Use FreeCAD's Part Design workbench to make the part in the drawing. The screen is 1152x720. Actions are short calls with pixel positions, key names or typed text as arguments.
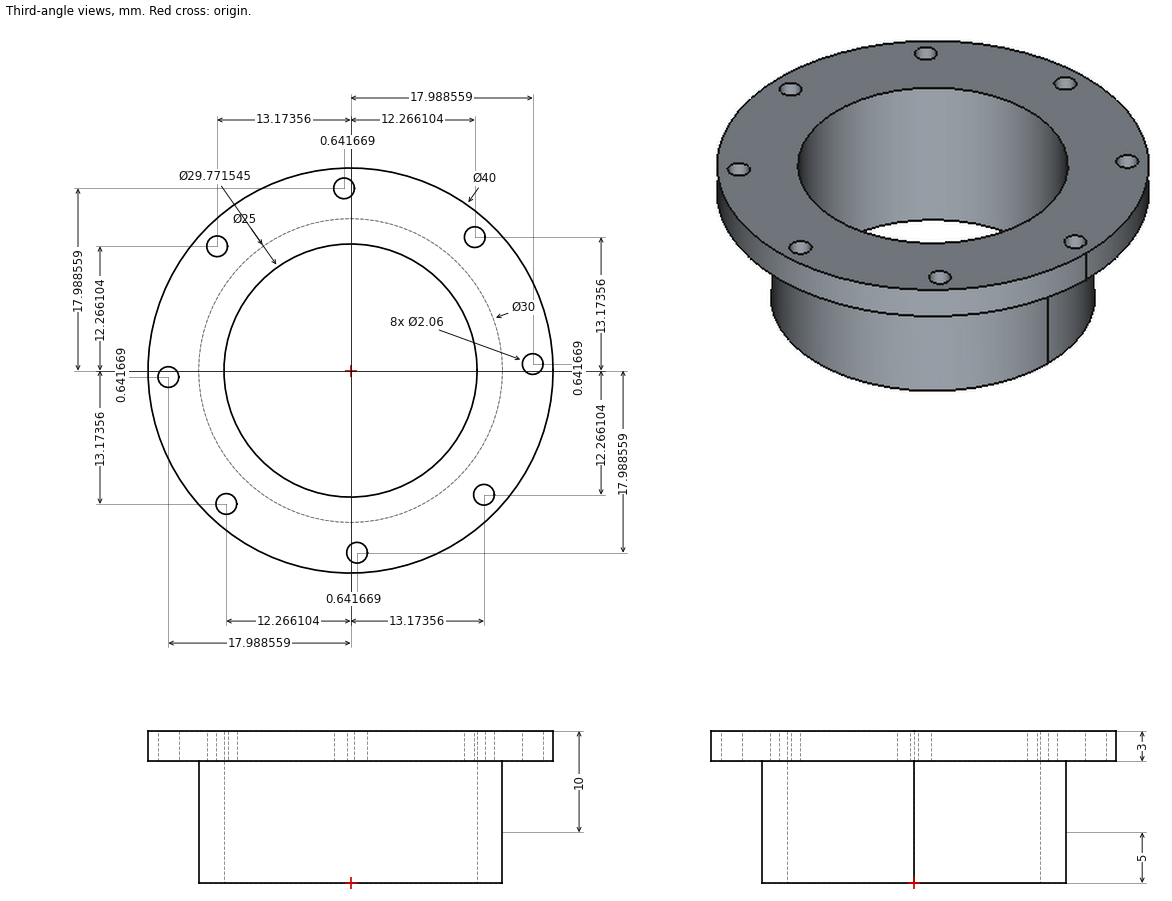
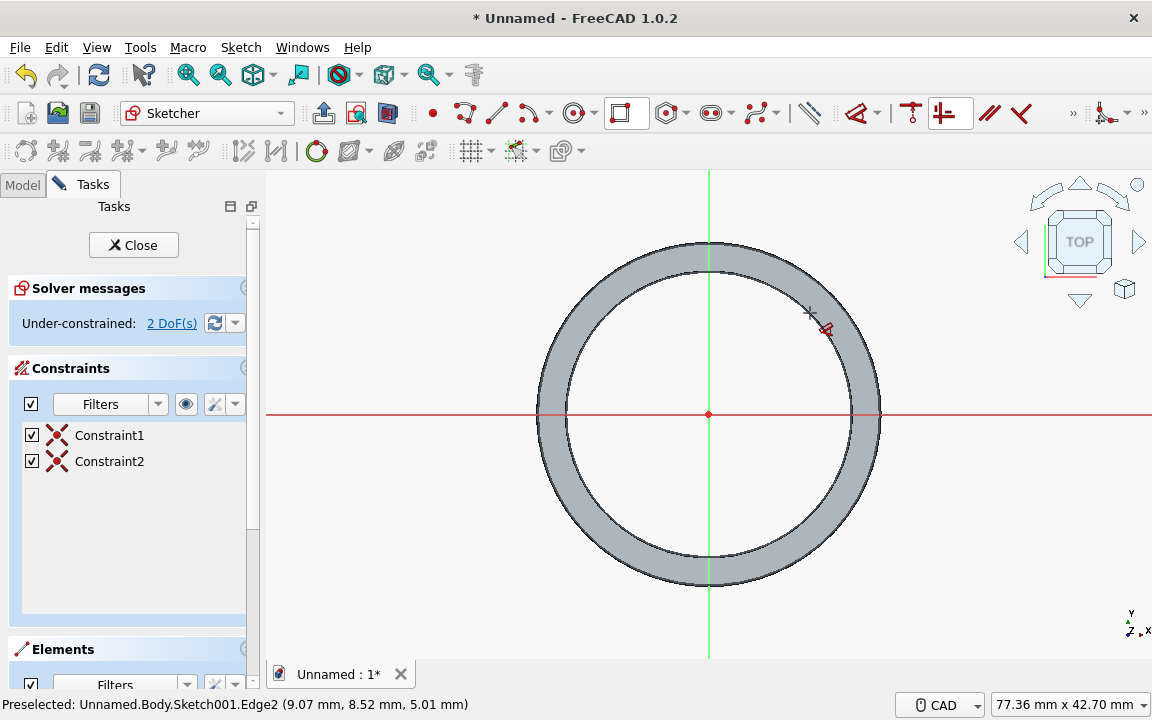
click(829, 293)
click(851, 270)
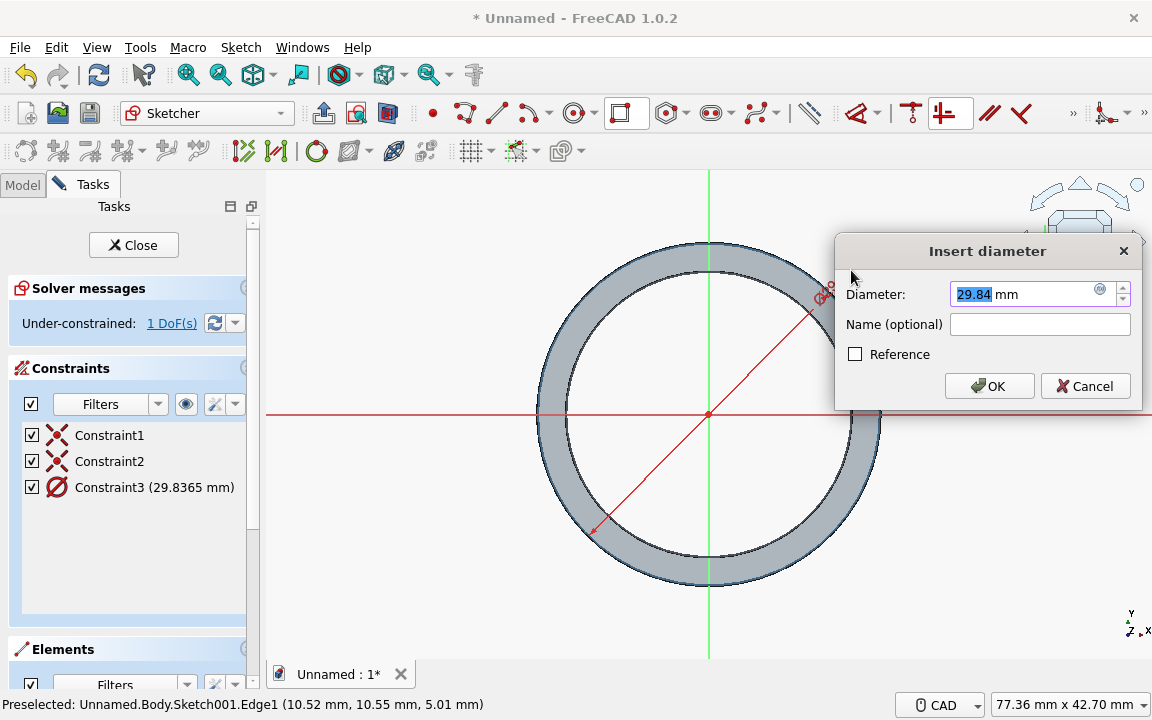
text(30)
key(Return)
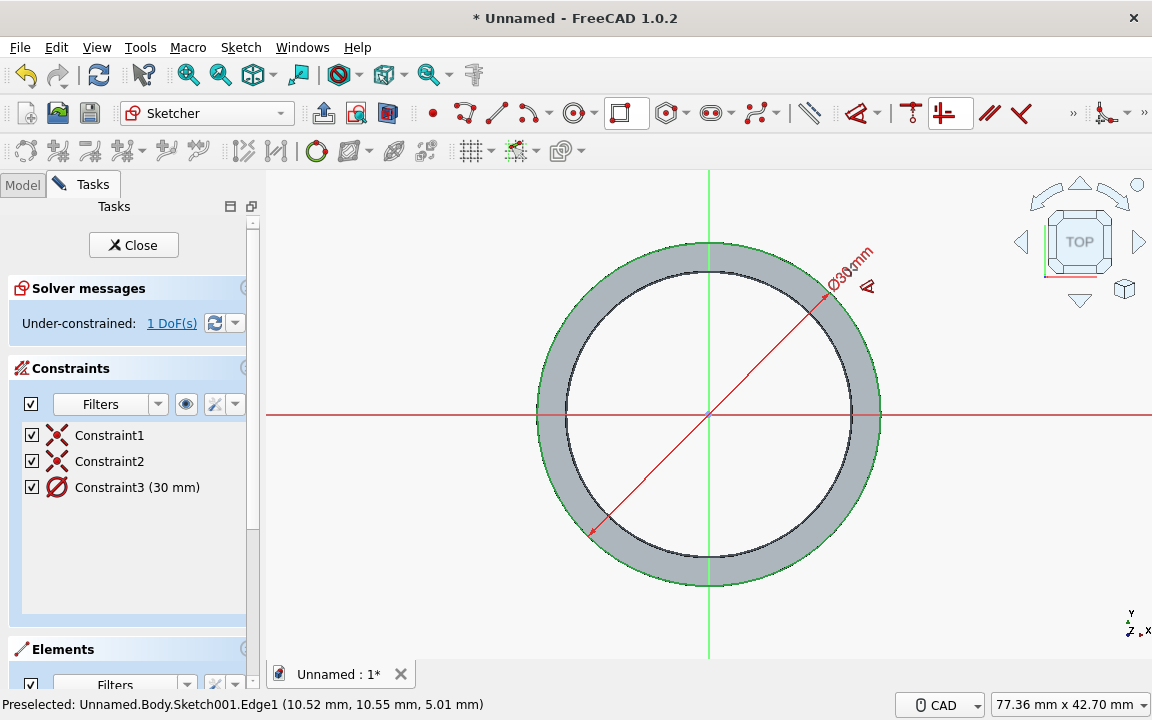
click(809, 313)
click(898, 358)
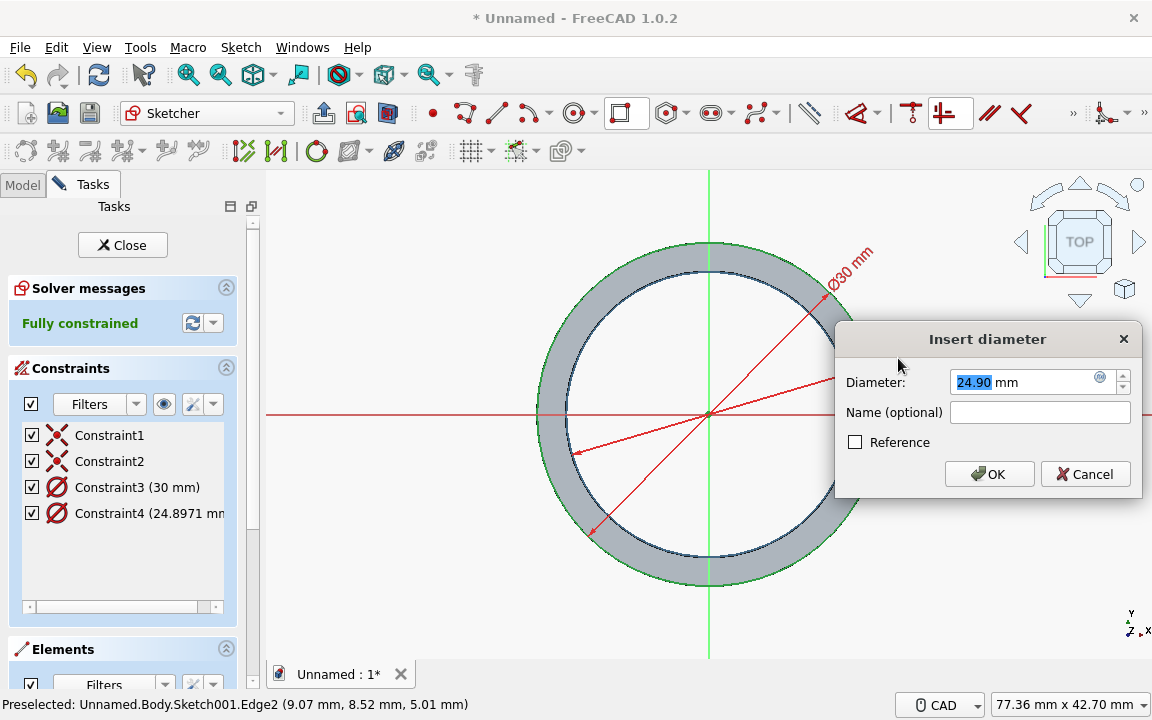
text(25)
key(Return)
key(Escape)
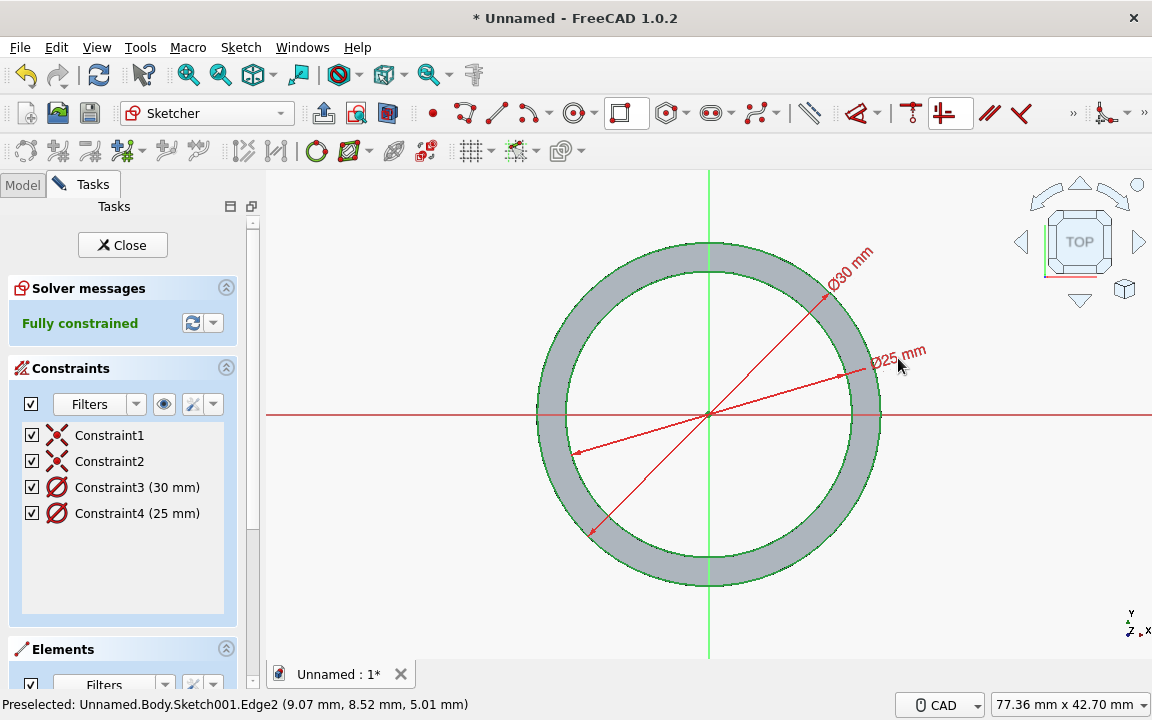
click(123, 245)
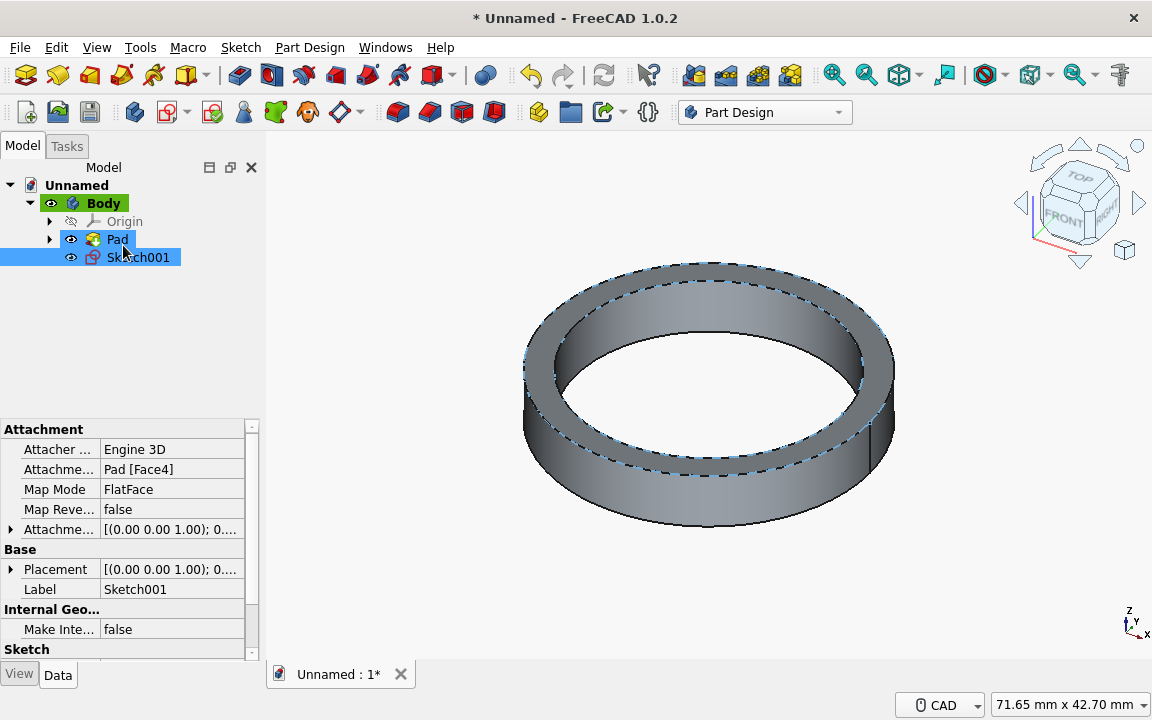
click(26, 76)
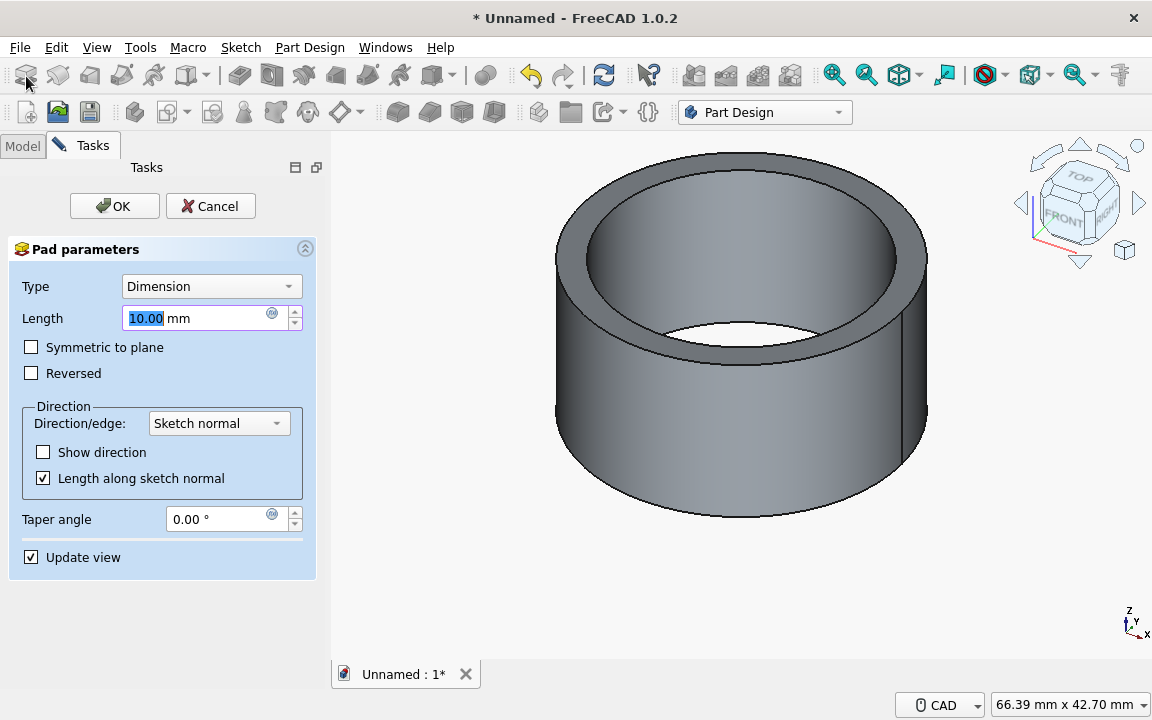
text(10)
key(Tab)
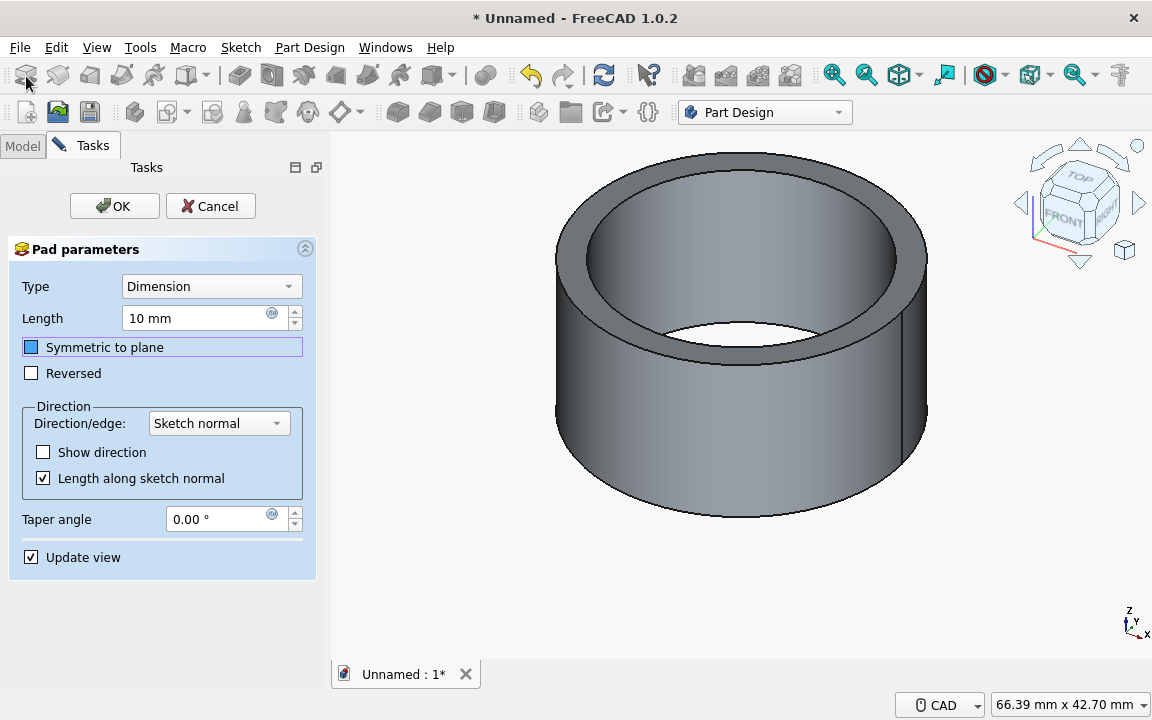
click(115, 206)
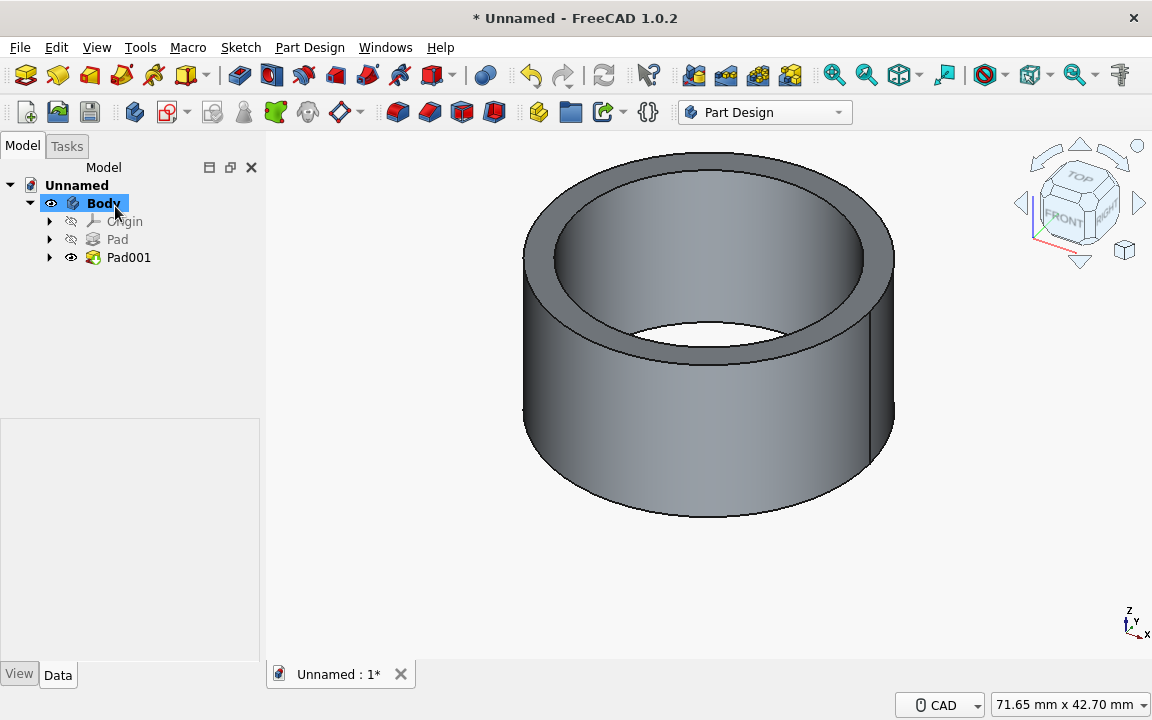
key(v)
key(f)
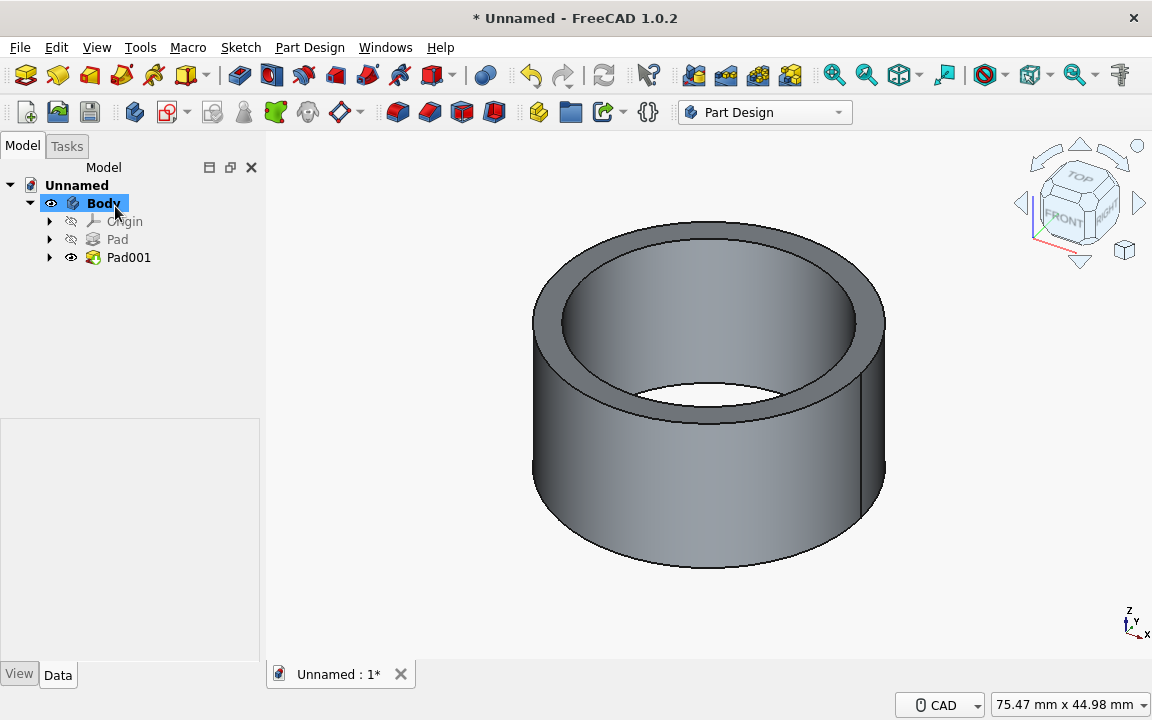
click(50, 221)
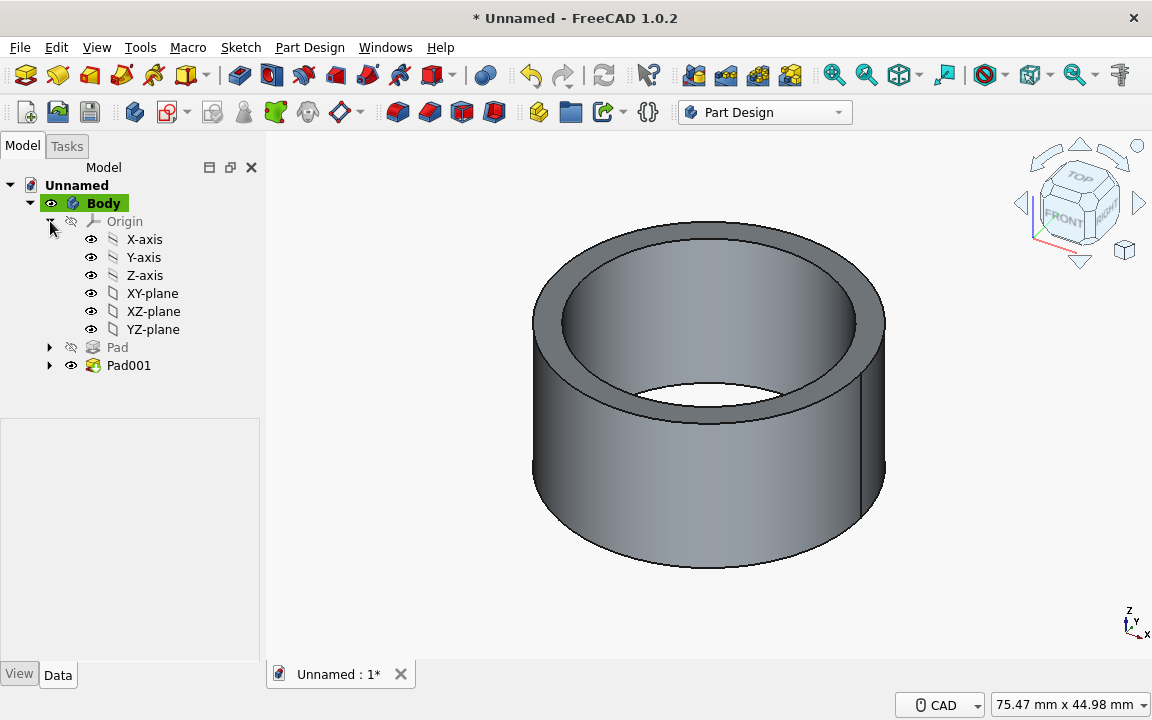
click(136, 293)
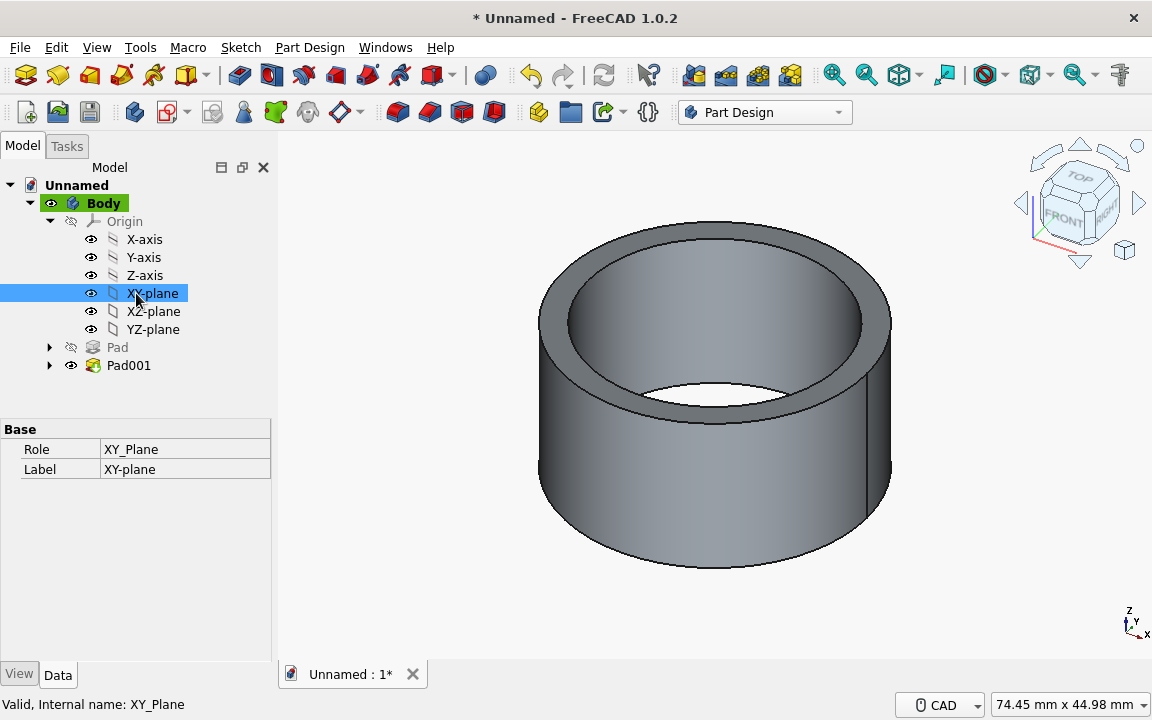
click(340, 112)